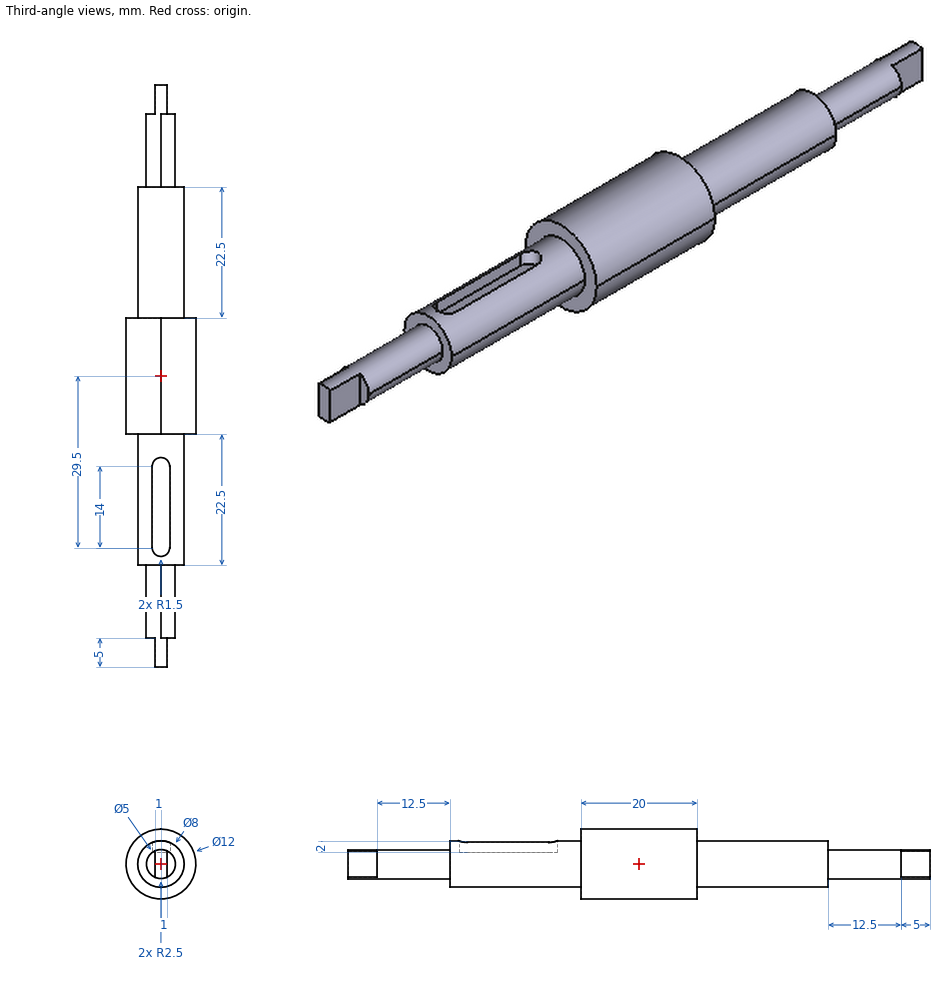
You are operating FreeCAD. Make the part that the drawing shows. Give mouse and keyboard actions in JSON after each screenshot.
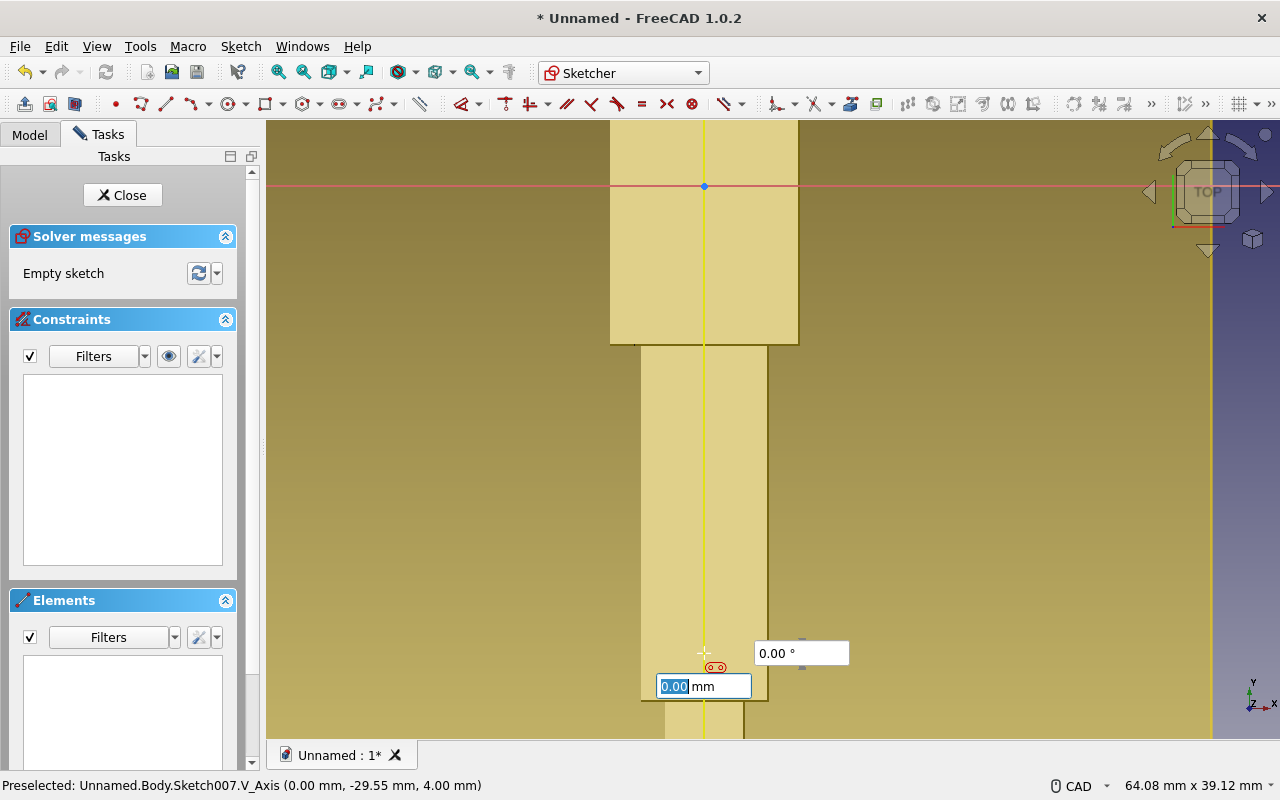
{"action": "left_click", "coordinate": [713, 432]}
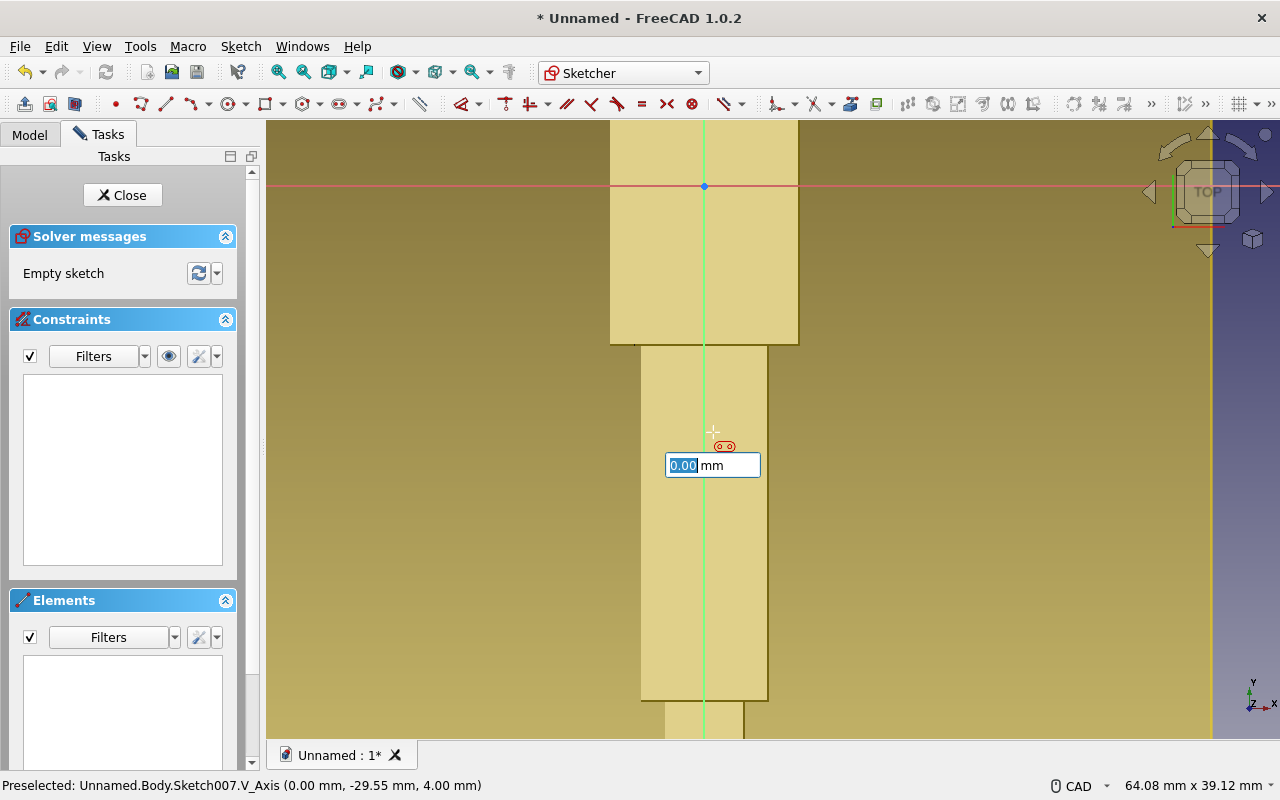
{"action": "left_click", "coordinate": [681, 542]}
{"action": "key", "text": "Escape"}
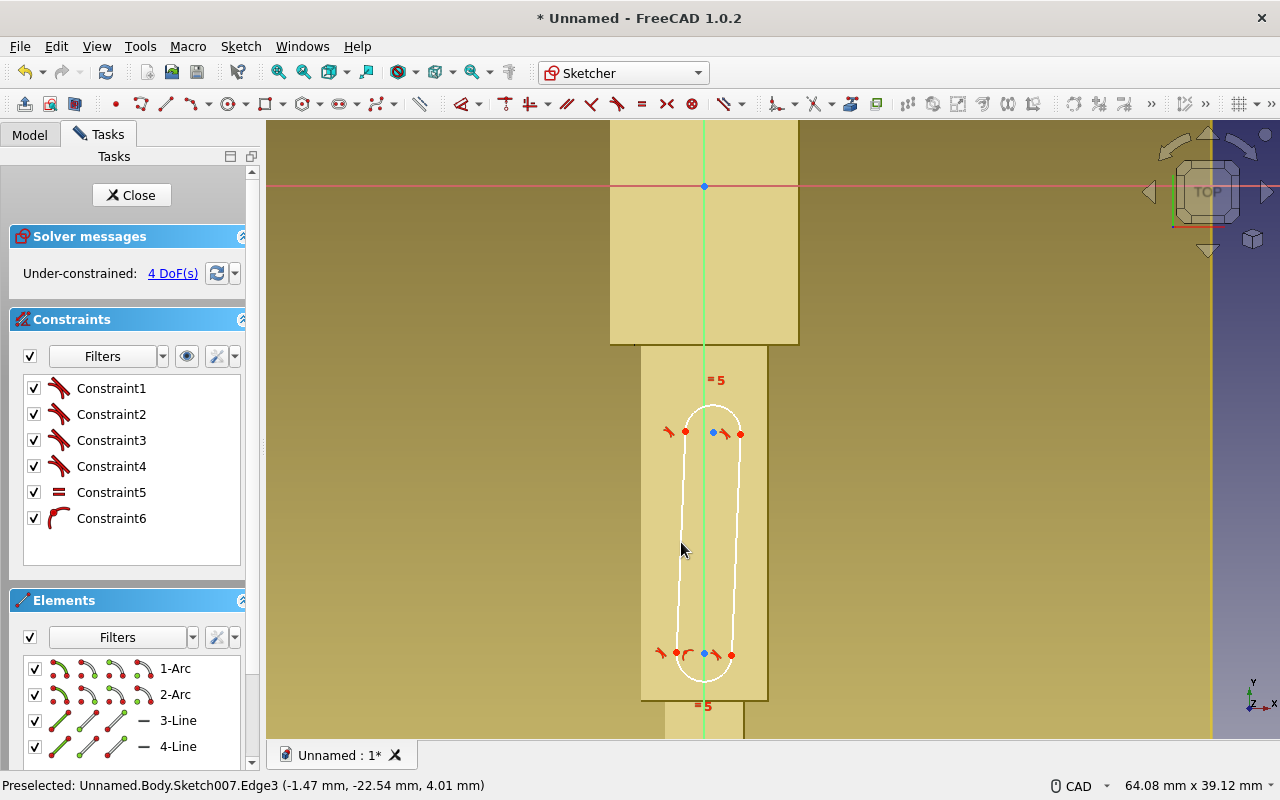
{"action": "left_click", "coordinate": [679, 587]}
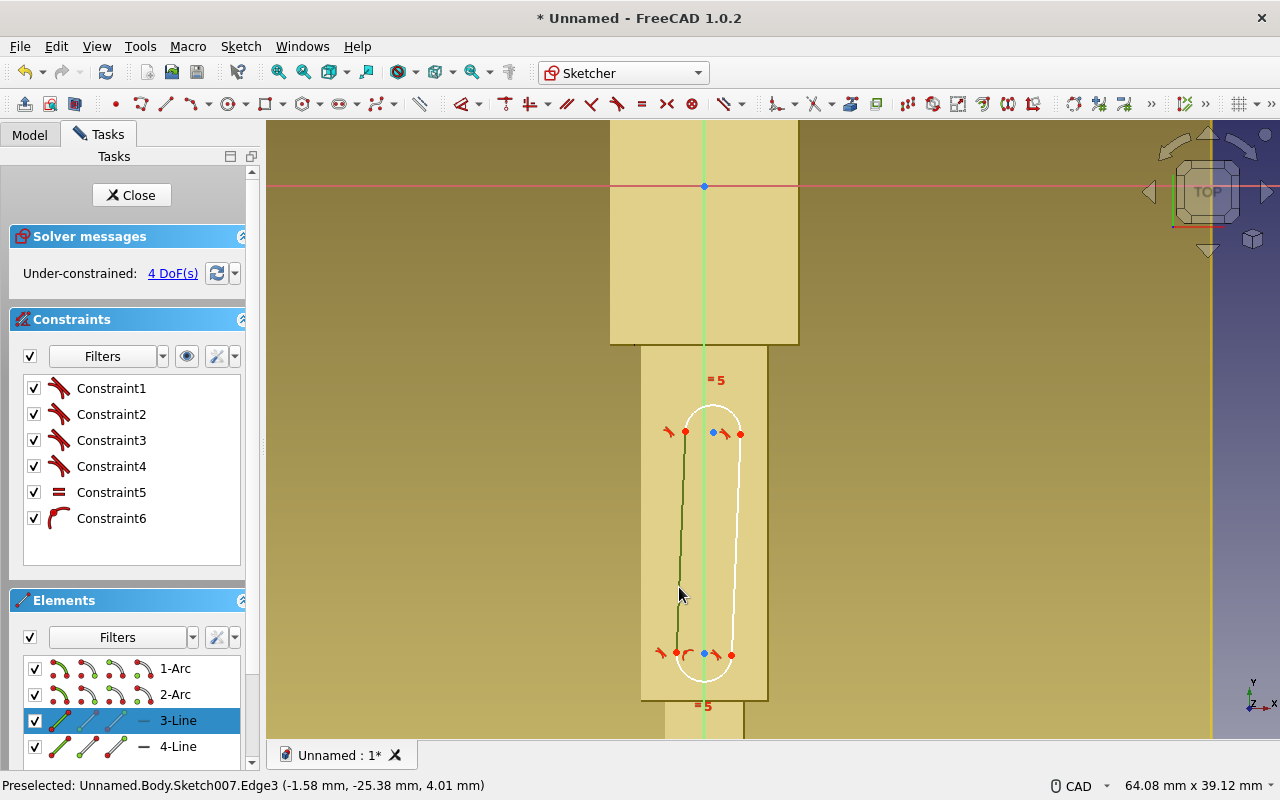
{"action": "key", "text": "v"}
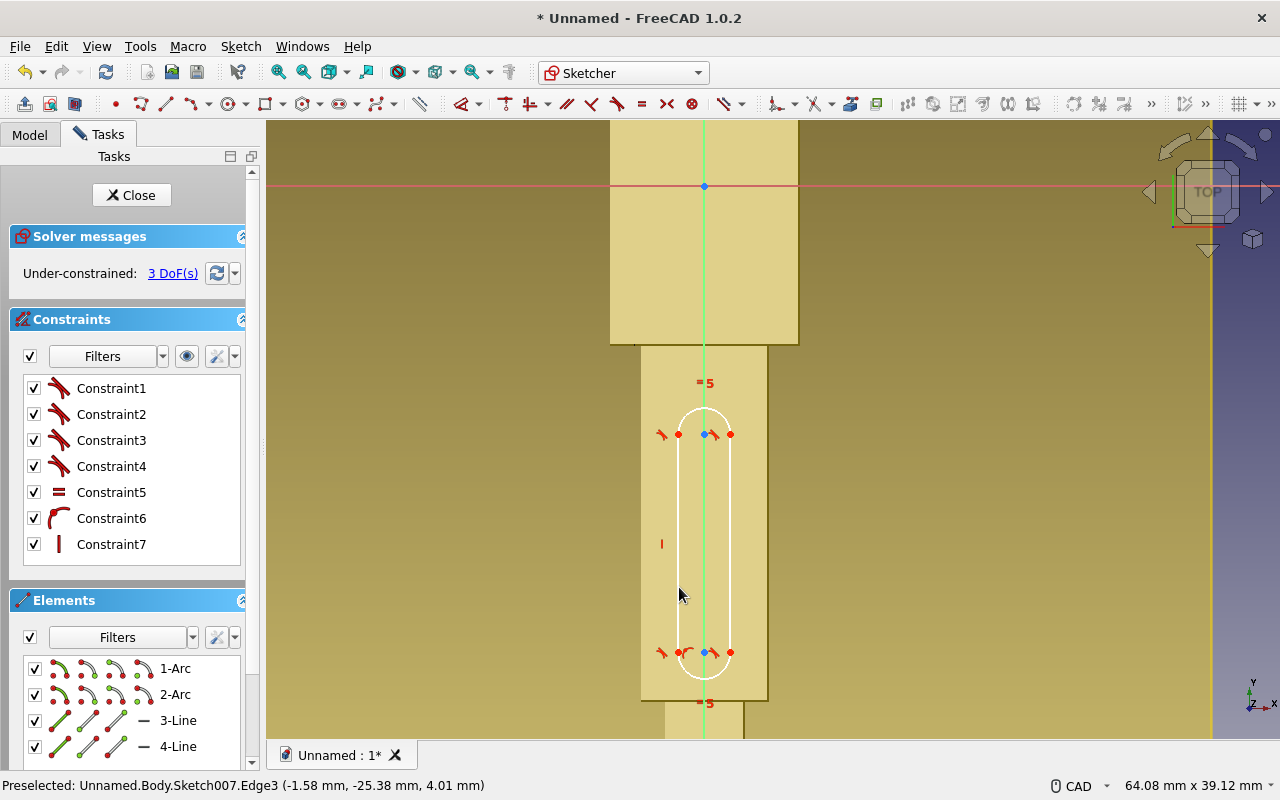
{"action": "key", "text": "d"}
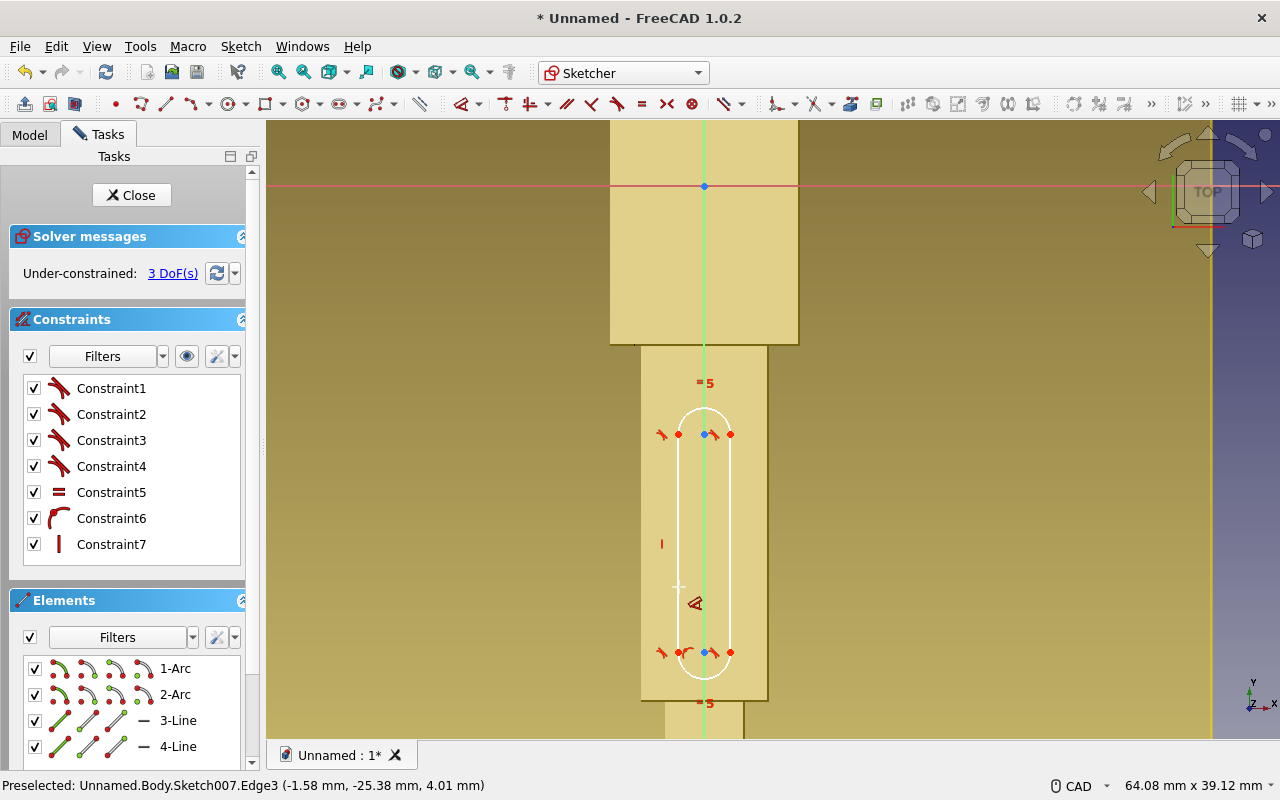
{"action": "scroll", "coordinate": [689, 674], "scroll_direction": "up", "scroll_amount": 3}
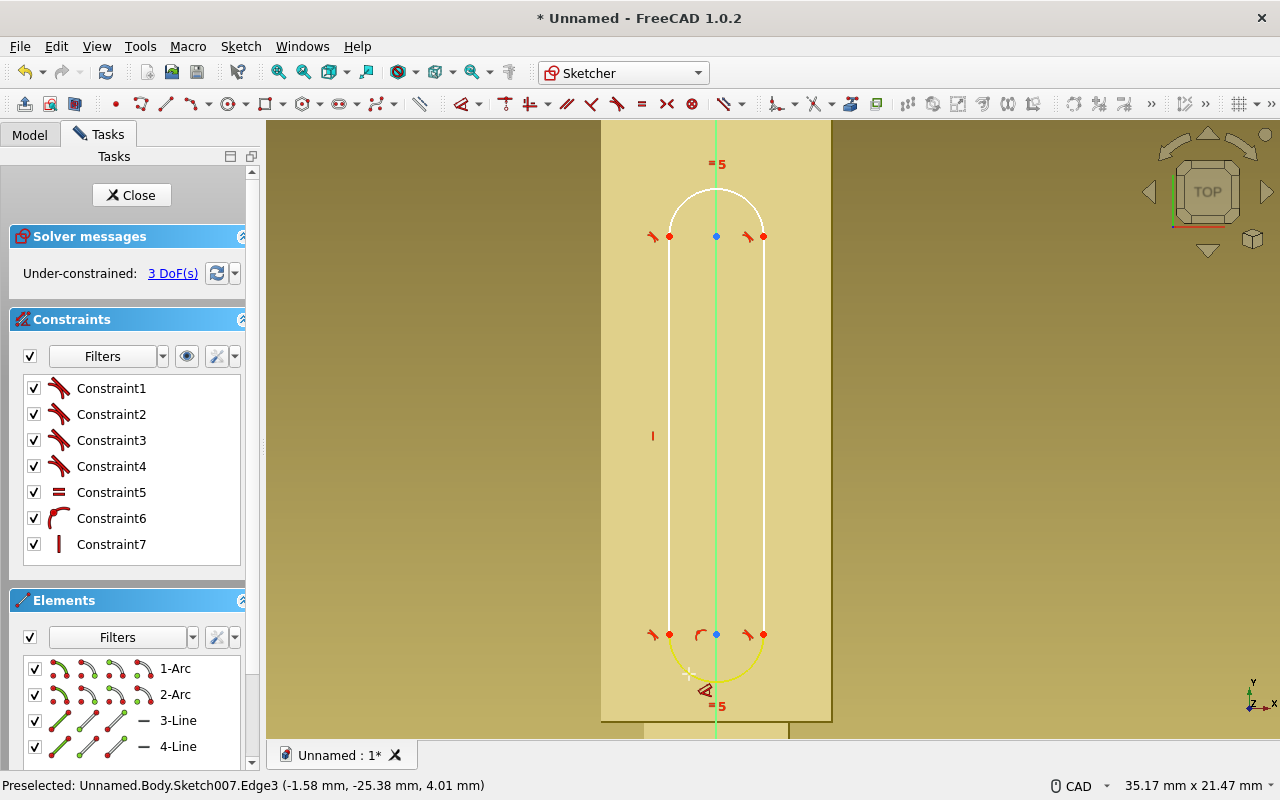
{"action": "left_click", "coordinate": [689, 673]}
{"action": "left_click", "coordinate": [670, 699]}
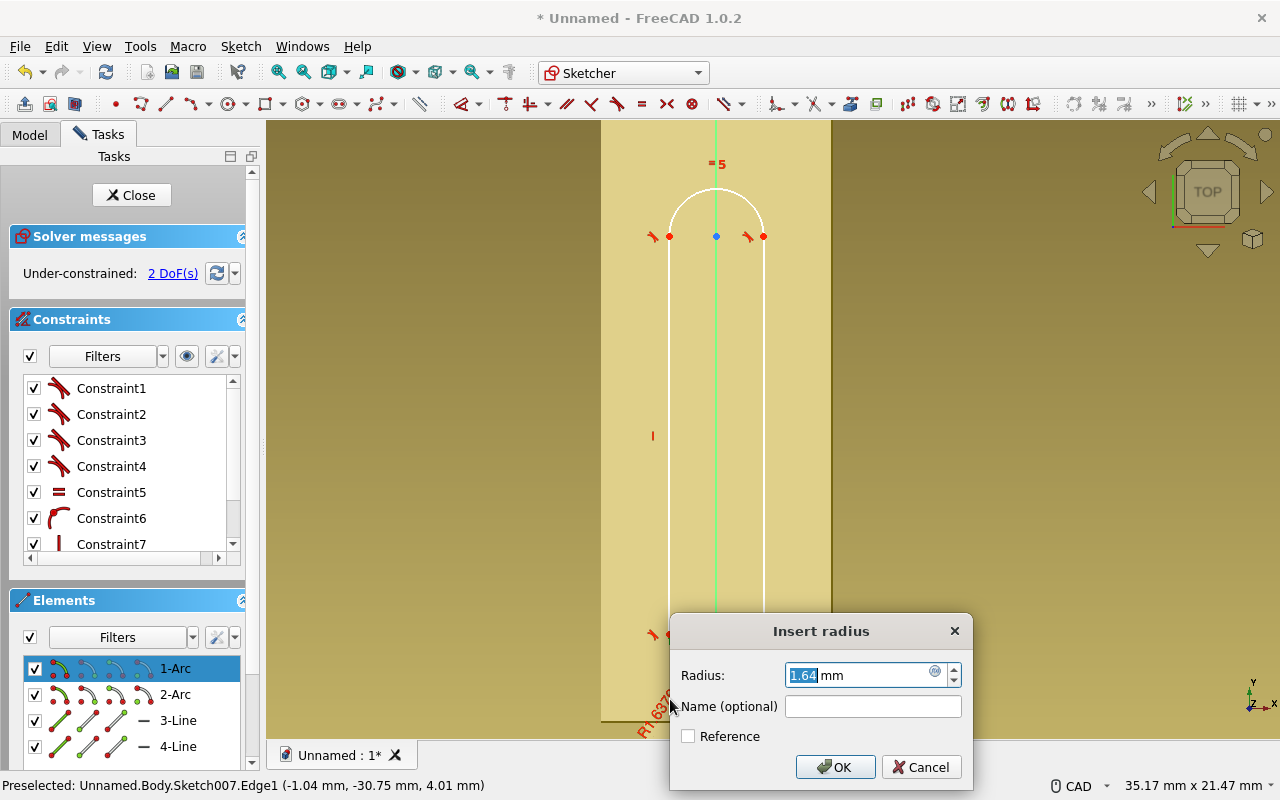
{"action": "type", "text": "1.5"}
{"action": "key", "text": "Return"}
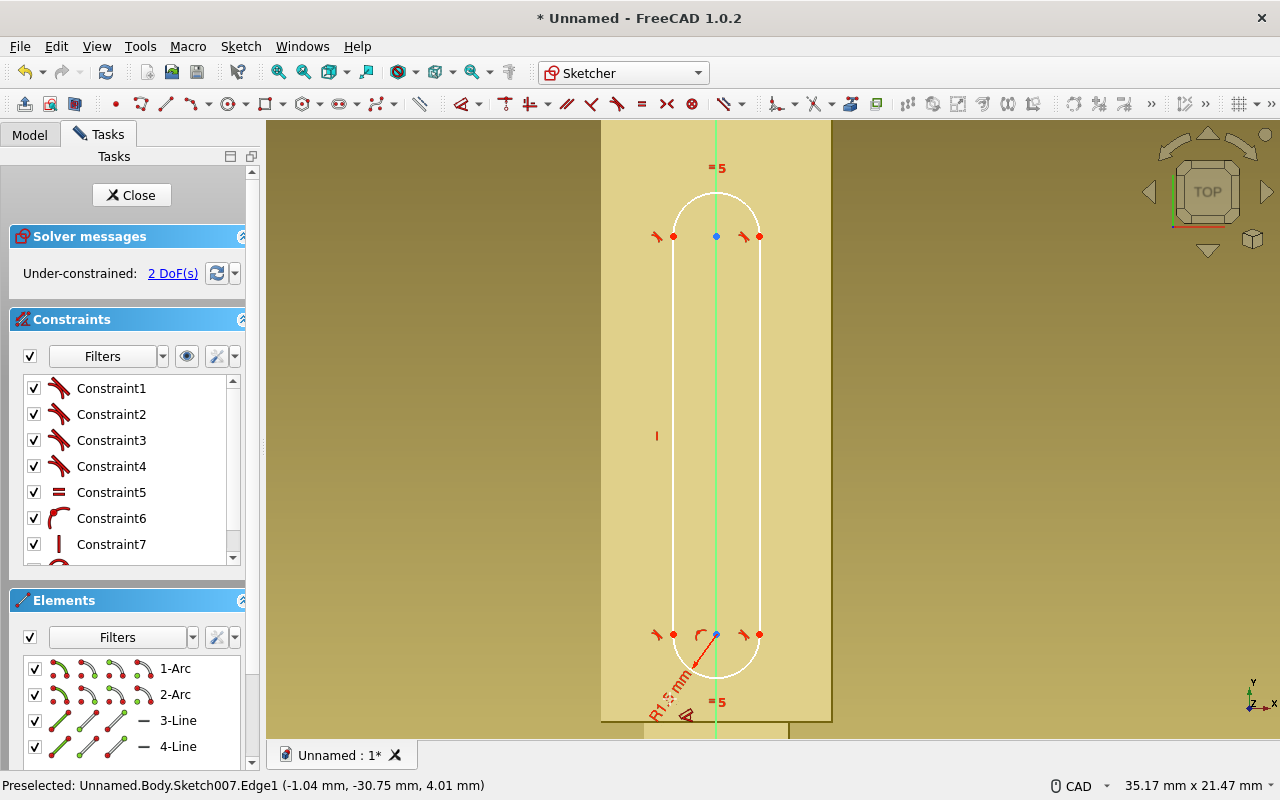
{"action": "left_click", "coordinate": [673, 515]}
{"action": "left_click", "coordinate": [639, 436]}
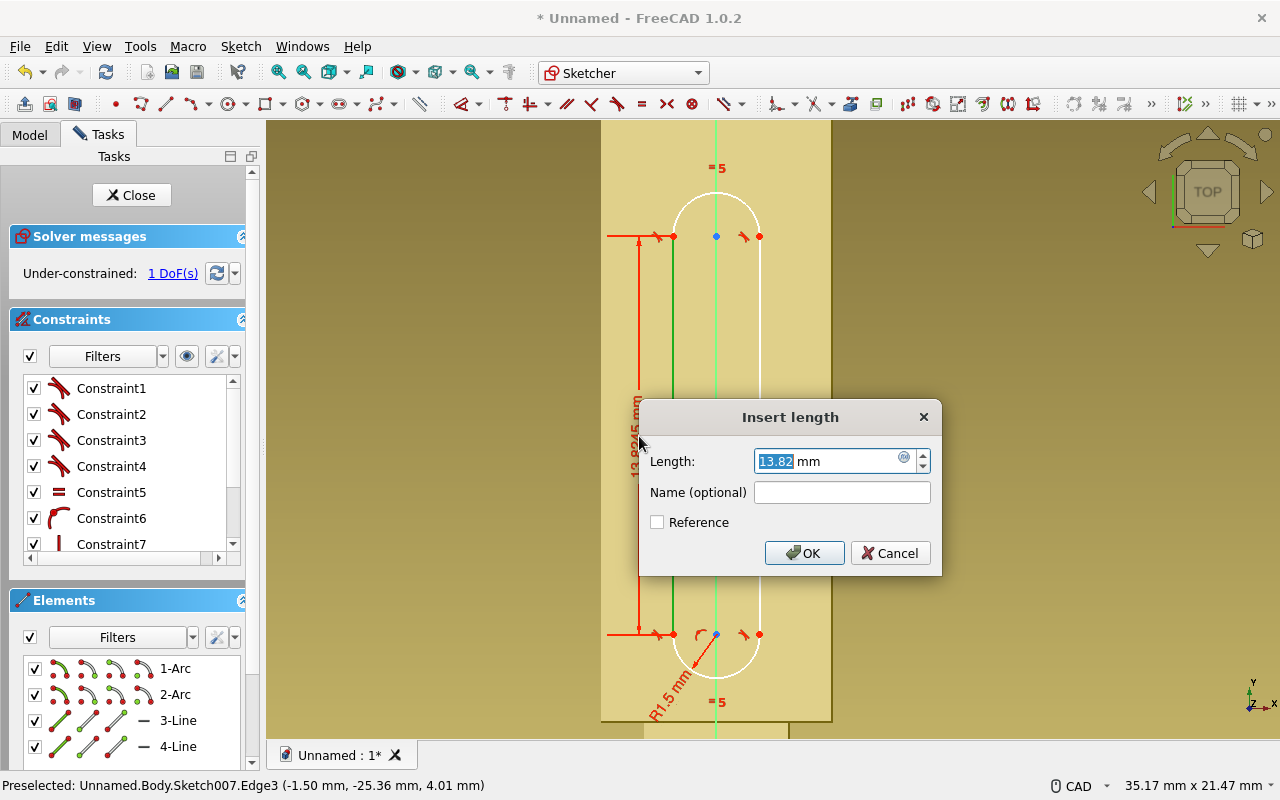
{"action": "type", "text": "14"}
{"action": "key", "text": "Return"}